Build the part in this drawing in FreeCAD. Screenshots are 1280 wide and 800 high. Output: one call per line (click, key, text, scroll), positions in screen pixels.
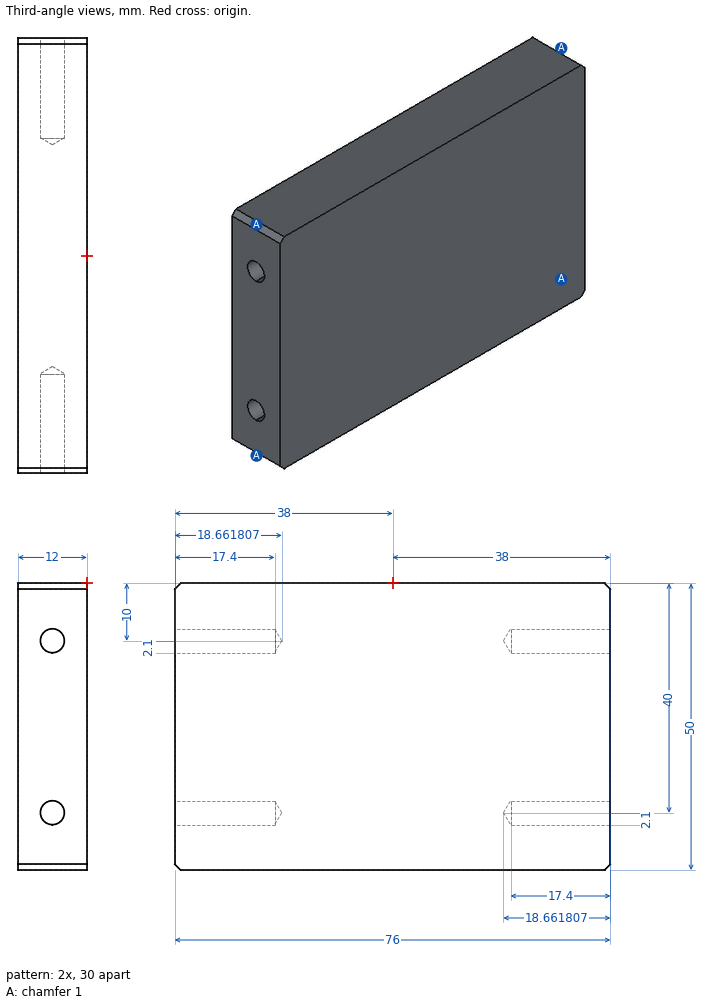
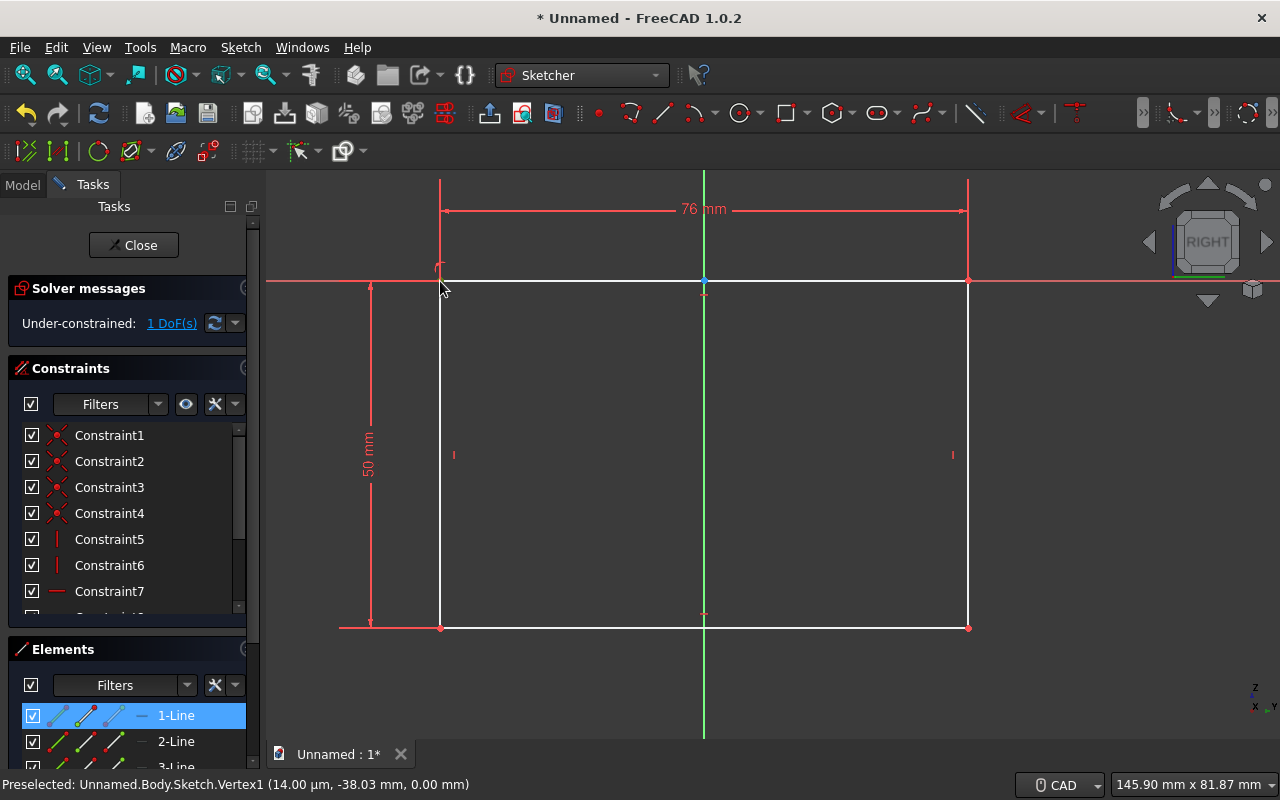
click(1044, 114)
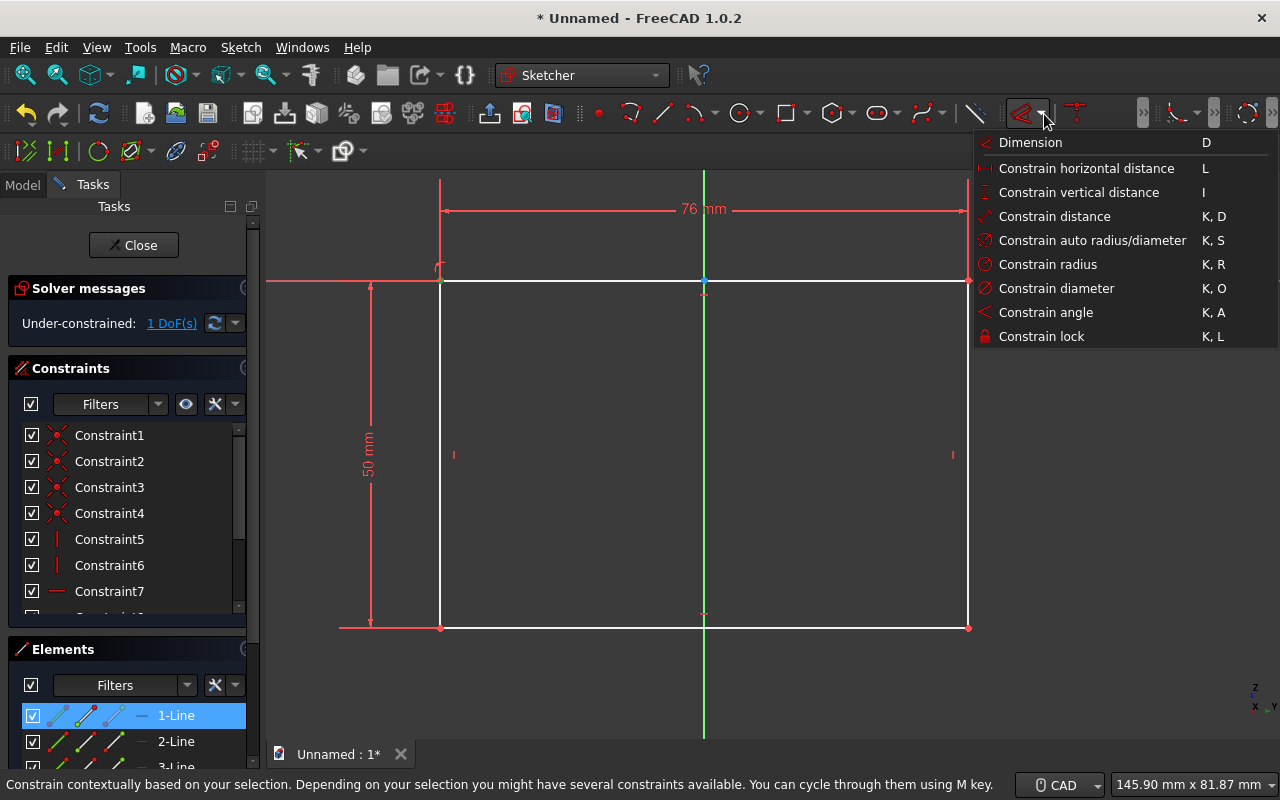
click(1126, 168)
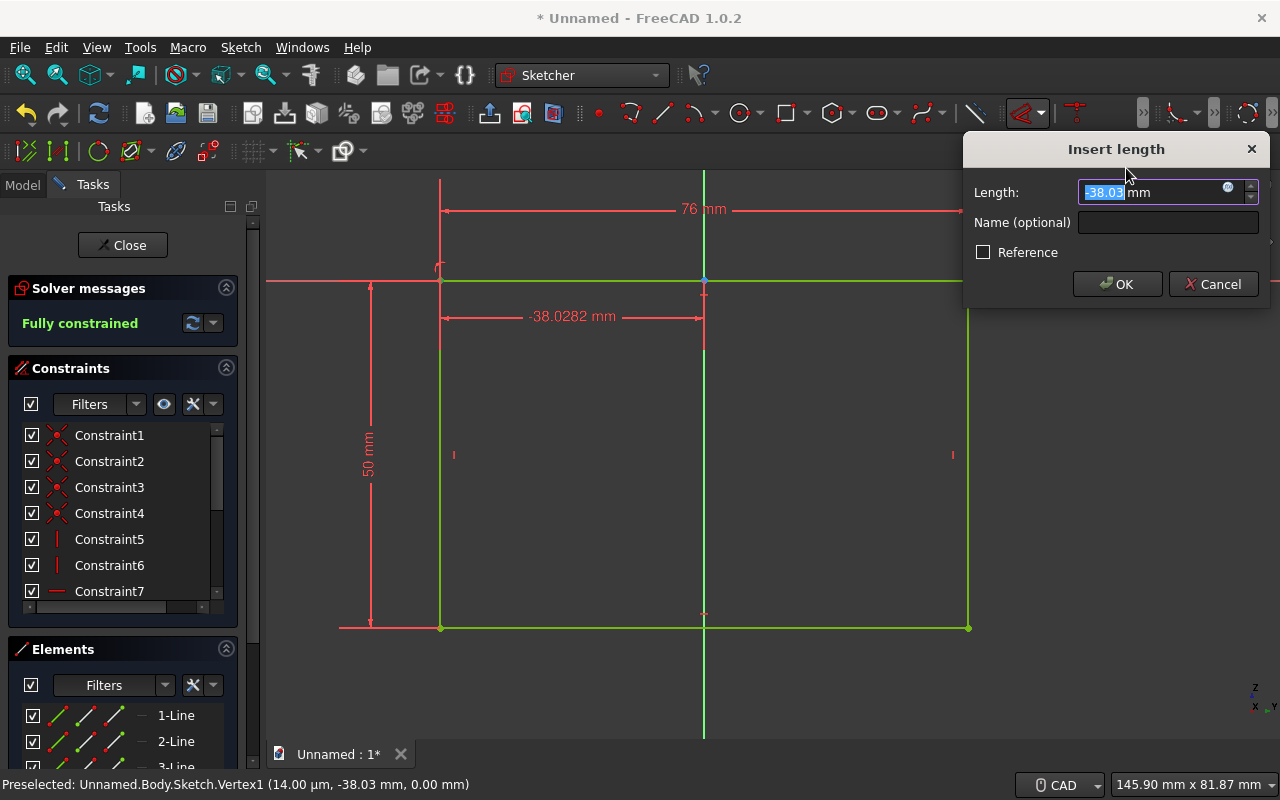
text(-38)
key(Return)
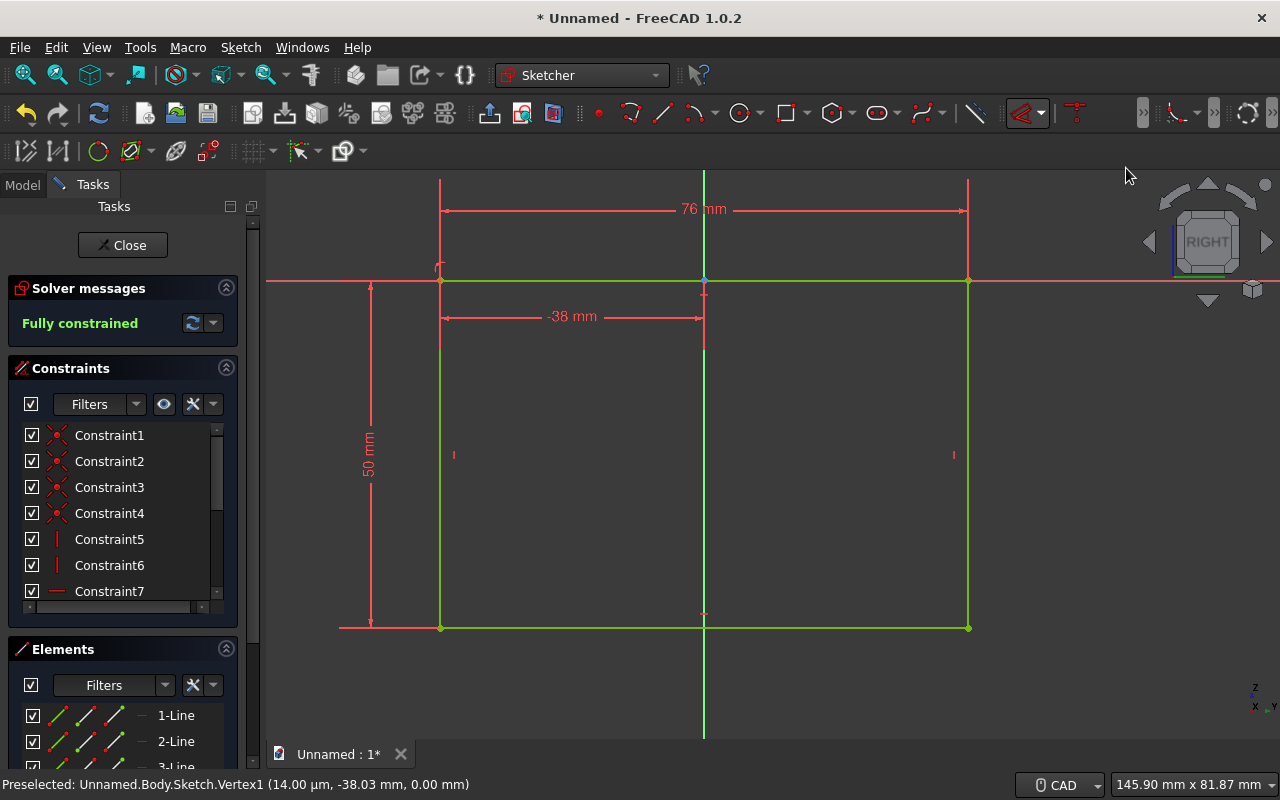
click(123, 245)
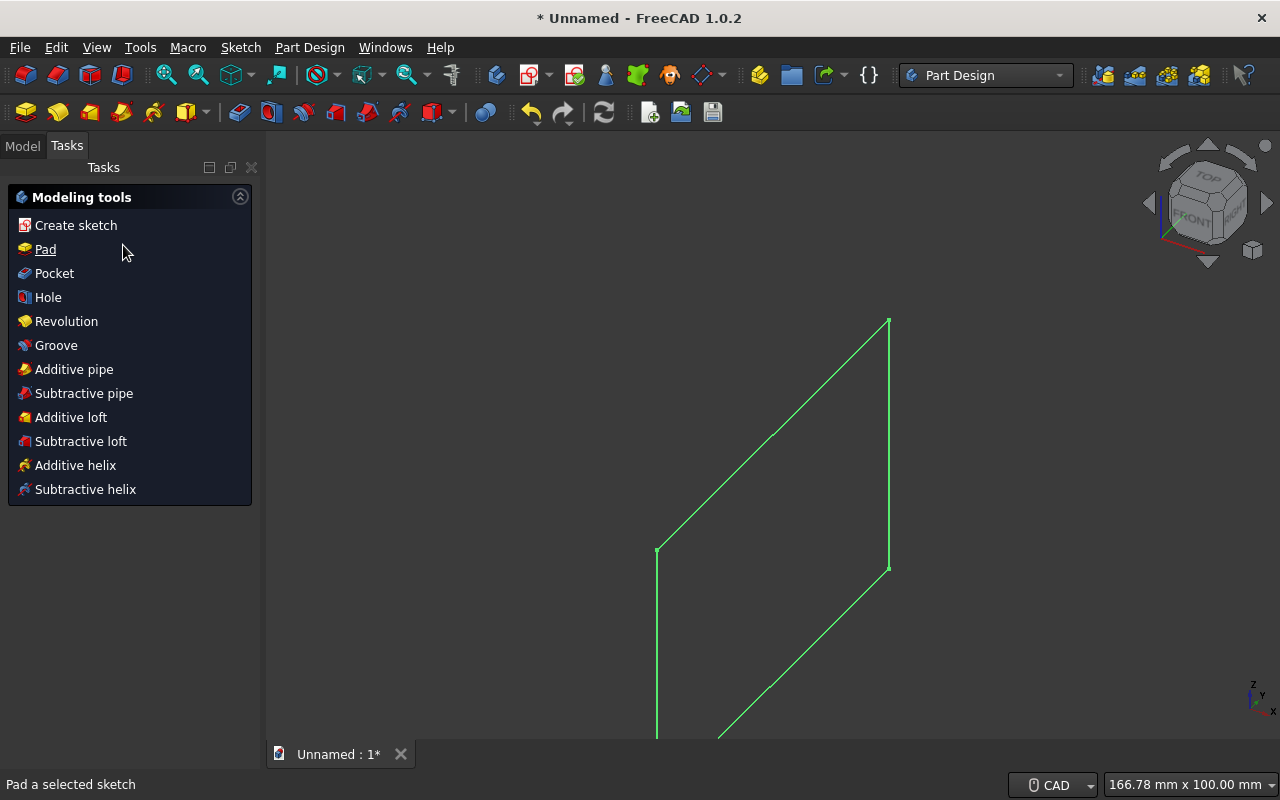
click(26, 112)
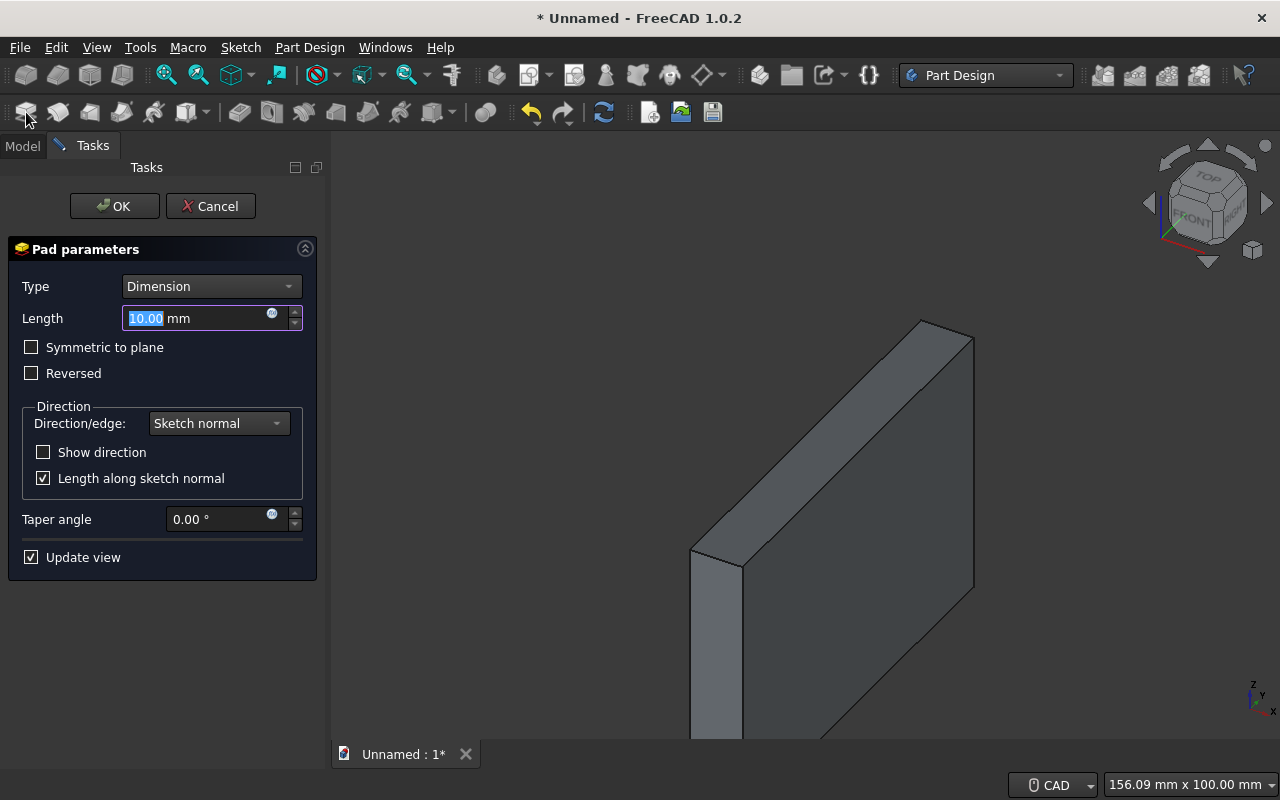
text(12)
key(Tab)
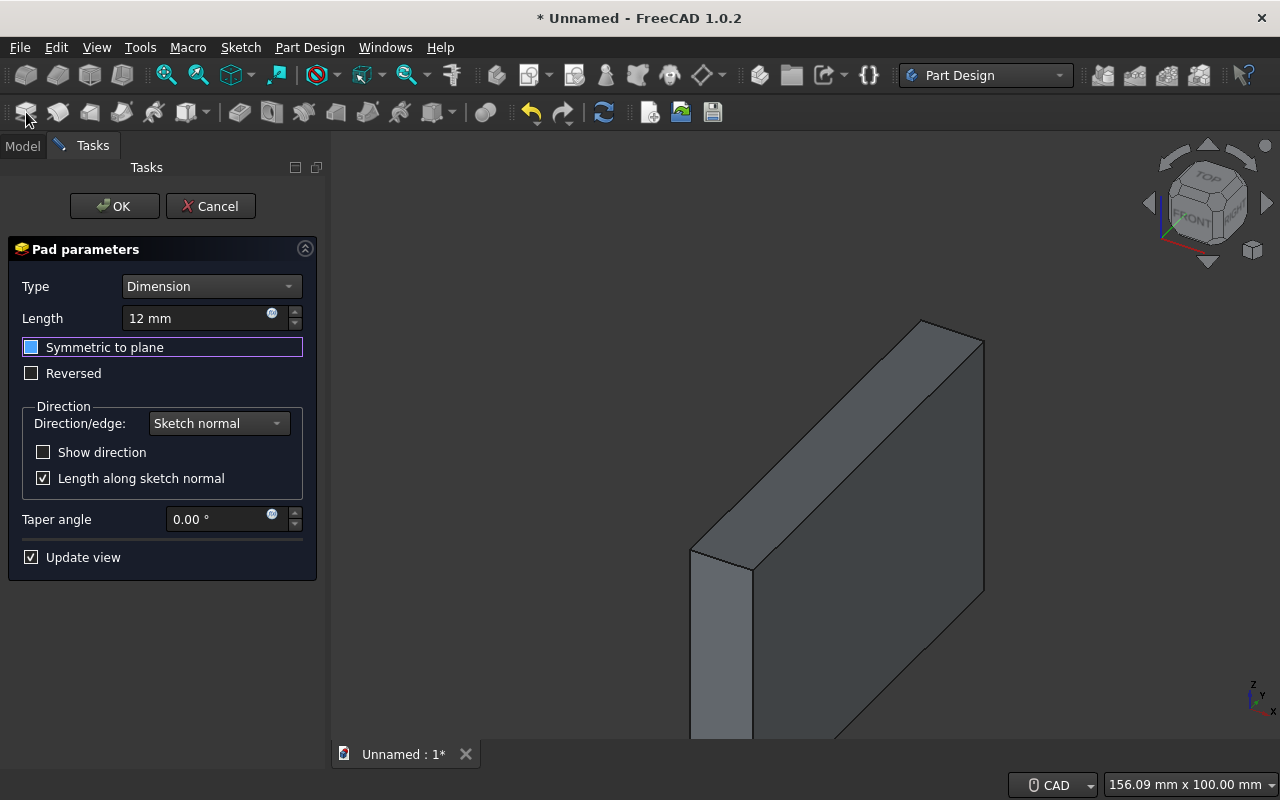
click(30, 373)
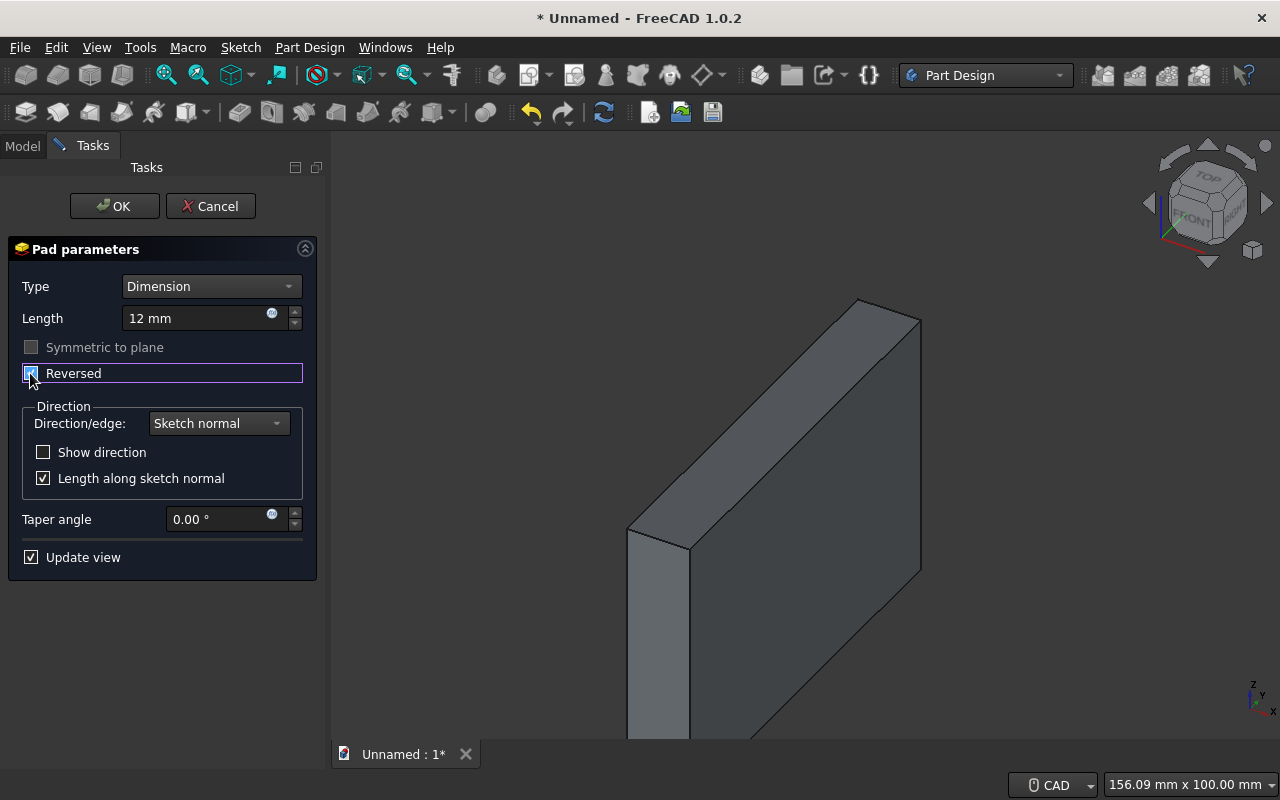
click(115, 206)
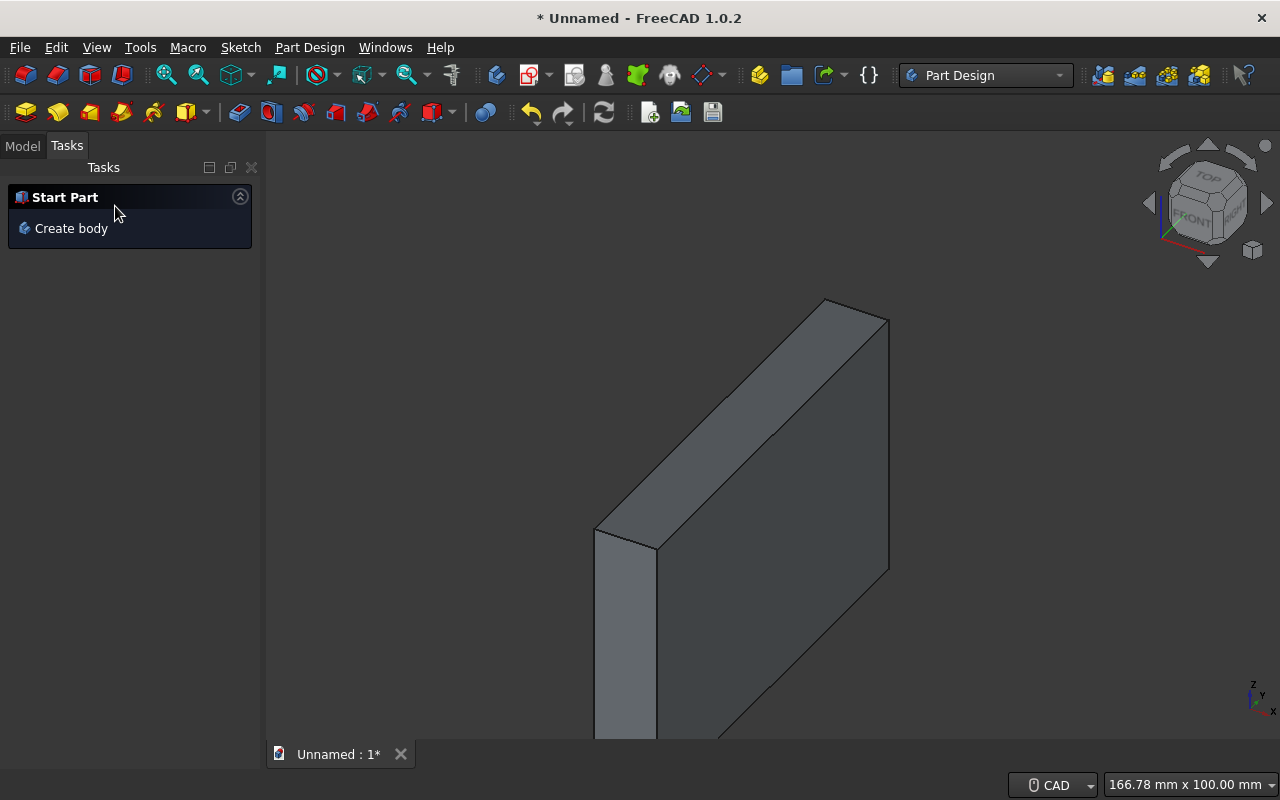
click(168, 76)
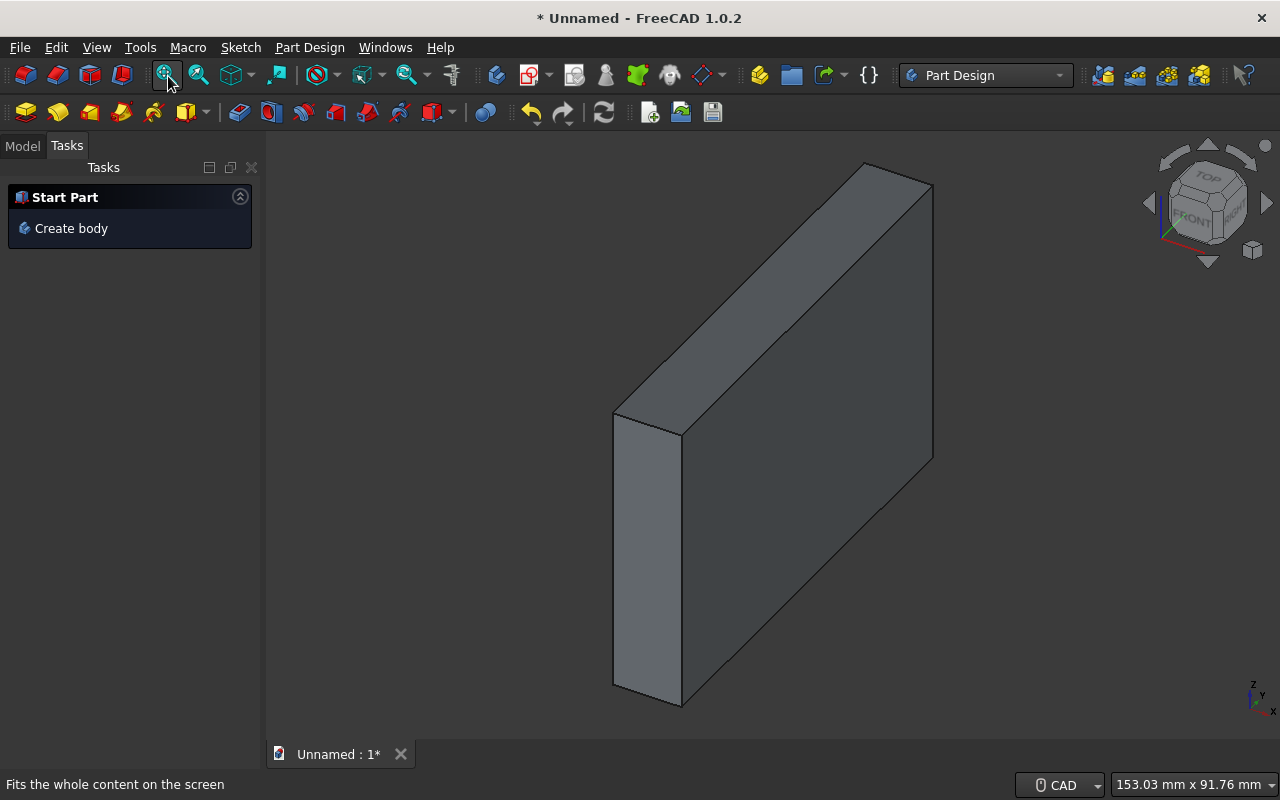
click(23, 145)